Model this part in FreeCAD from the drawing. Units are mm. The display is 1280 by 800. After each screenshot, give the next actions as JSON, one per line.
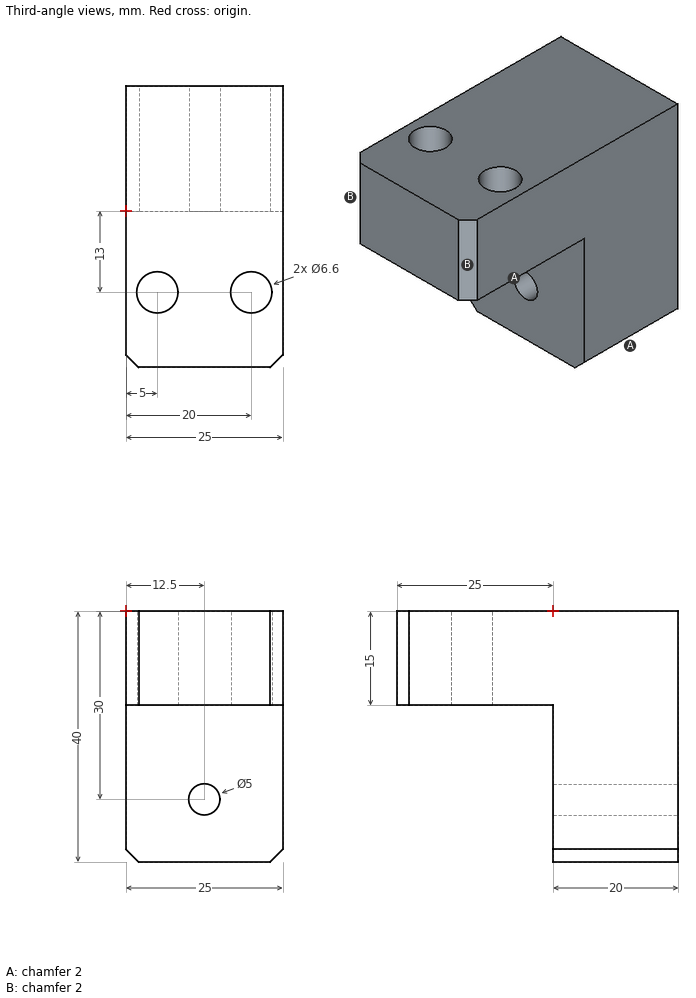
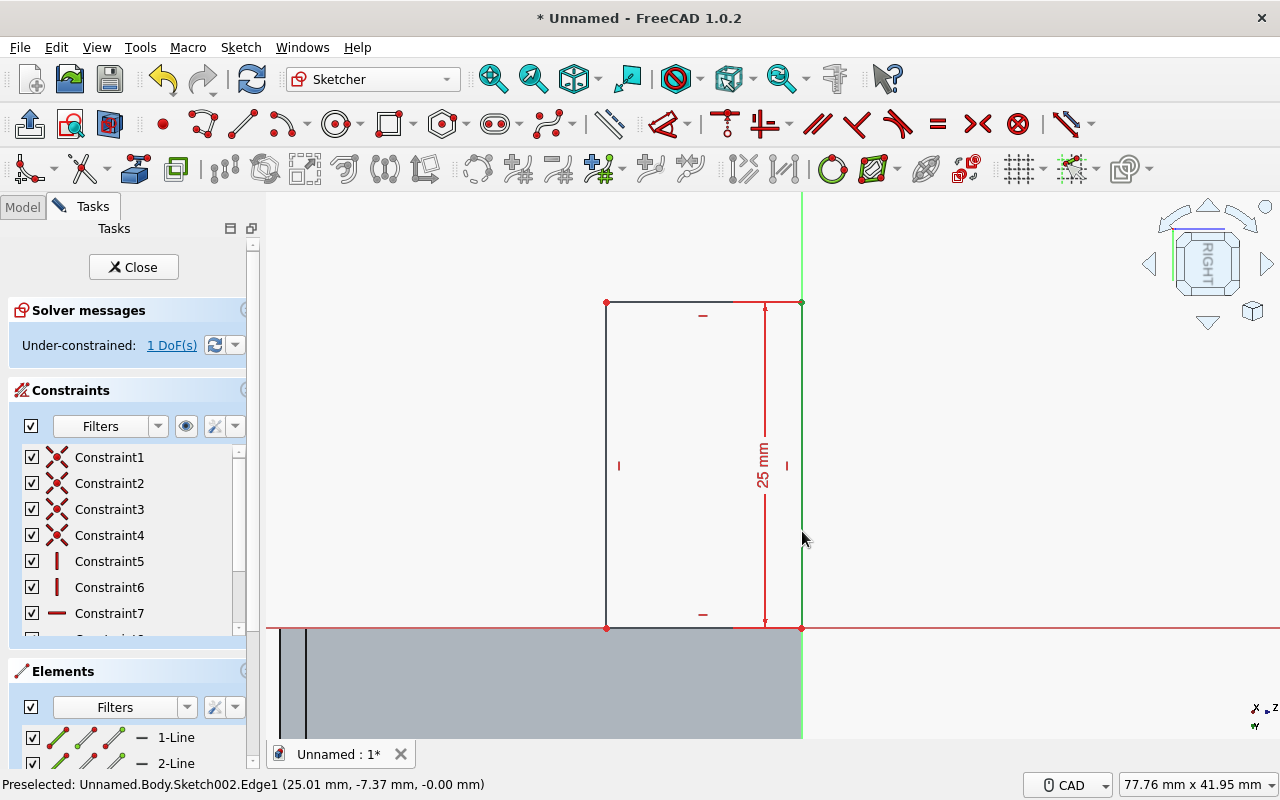
{"action": "left_click", "coordinate": [743, 302]}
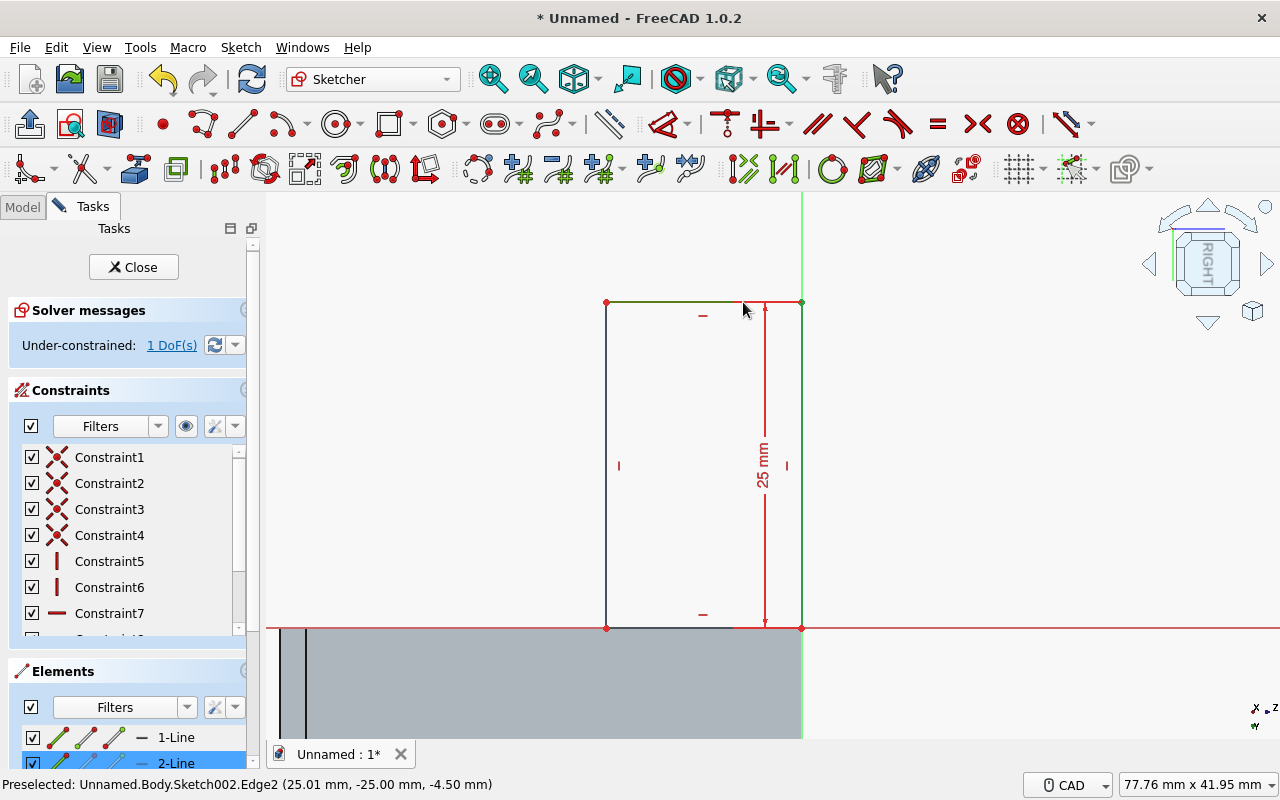
{"action": "left_click", "coordinate": [690, 124]}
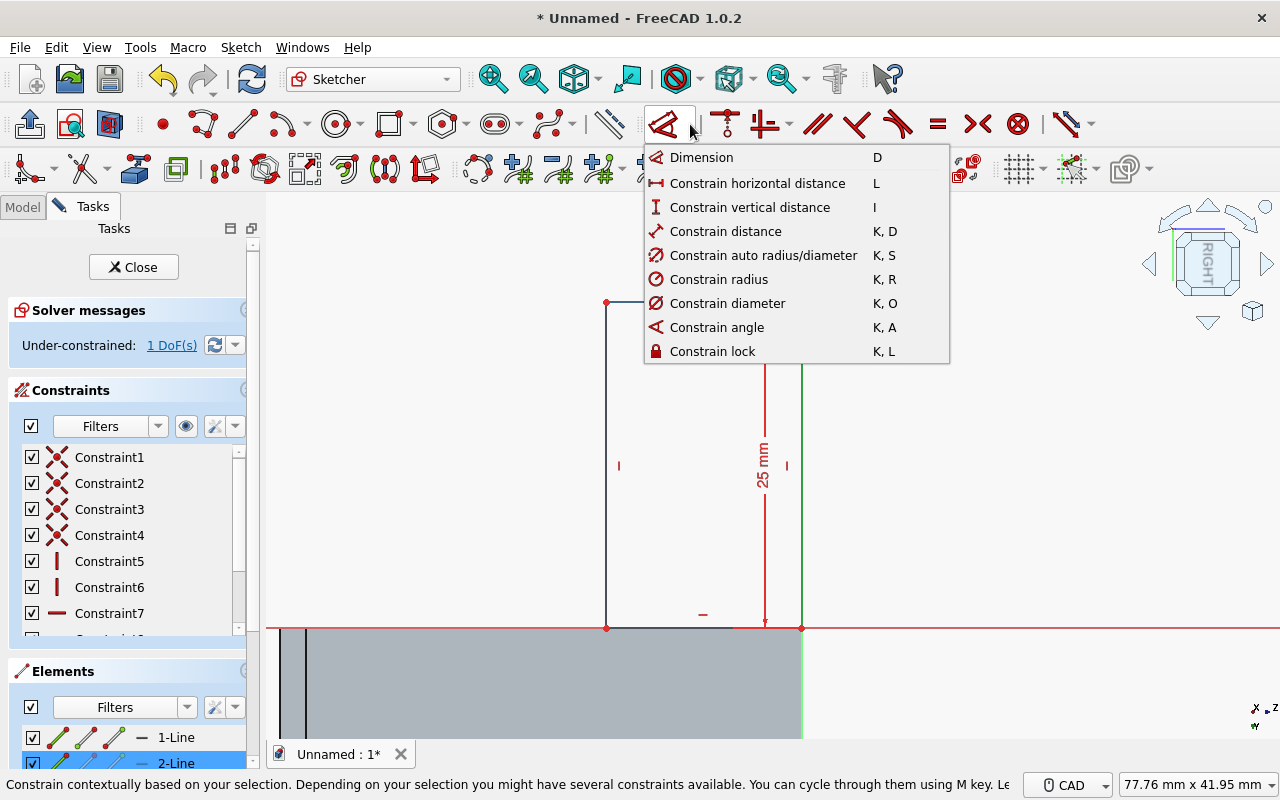
{"action": "left_click", "coordinate": [797, 183]}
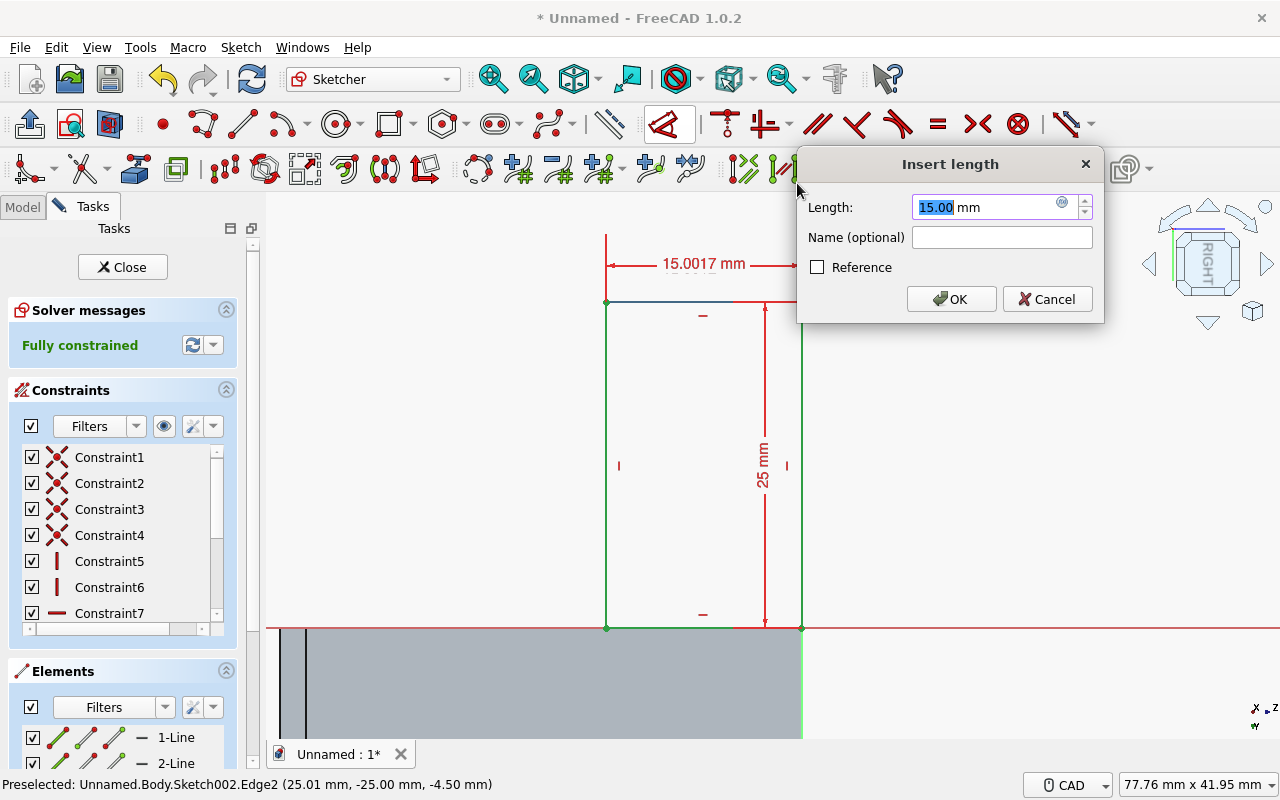
{"action": "type", "text": "15"}
{"action": "key", "text": "Return"}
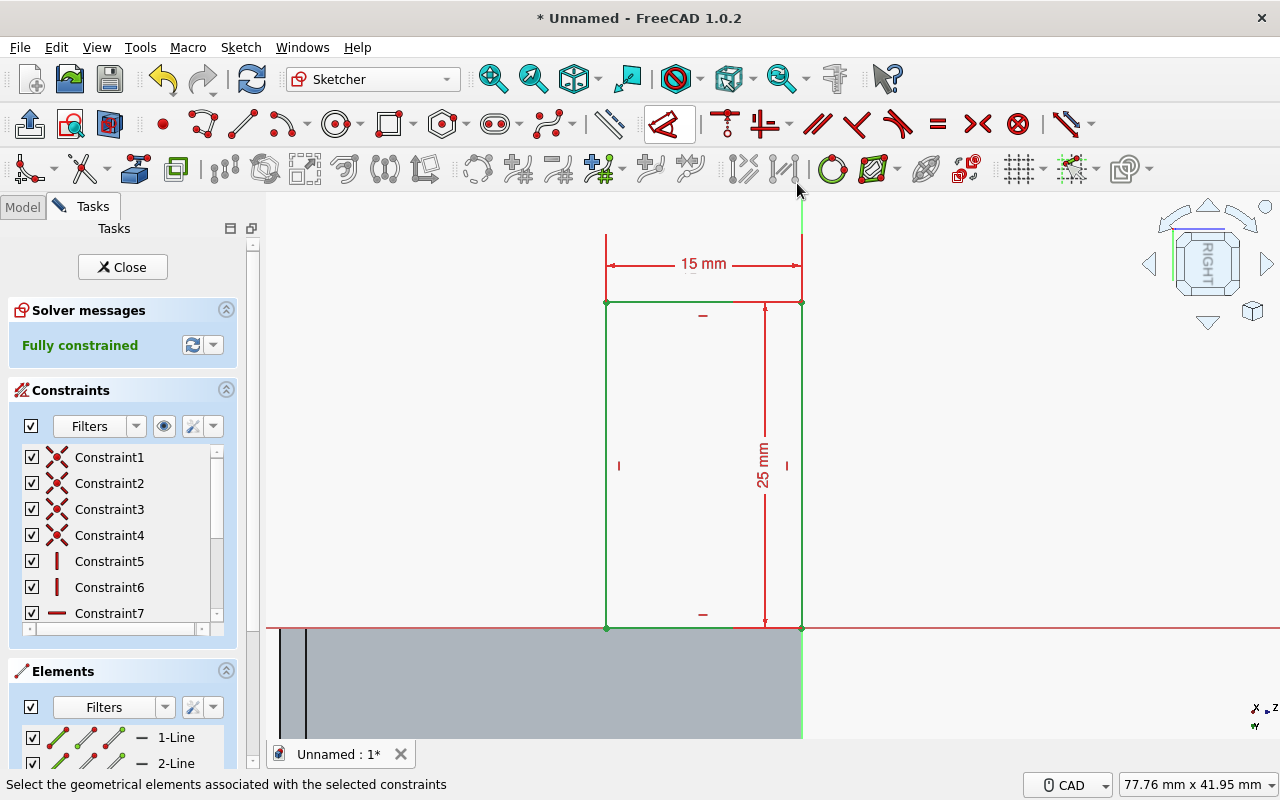
{"action": "left_click", "coordinate": [123, 267]}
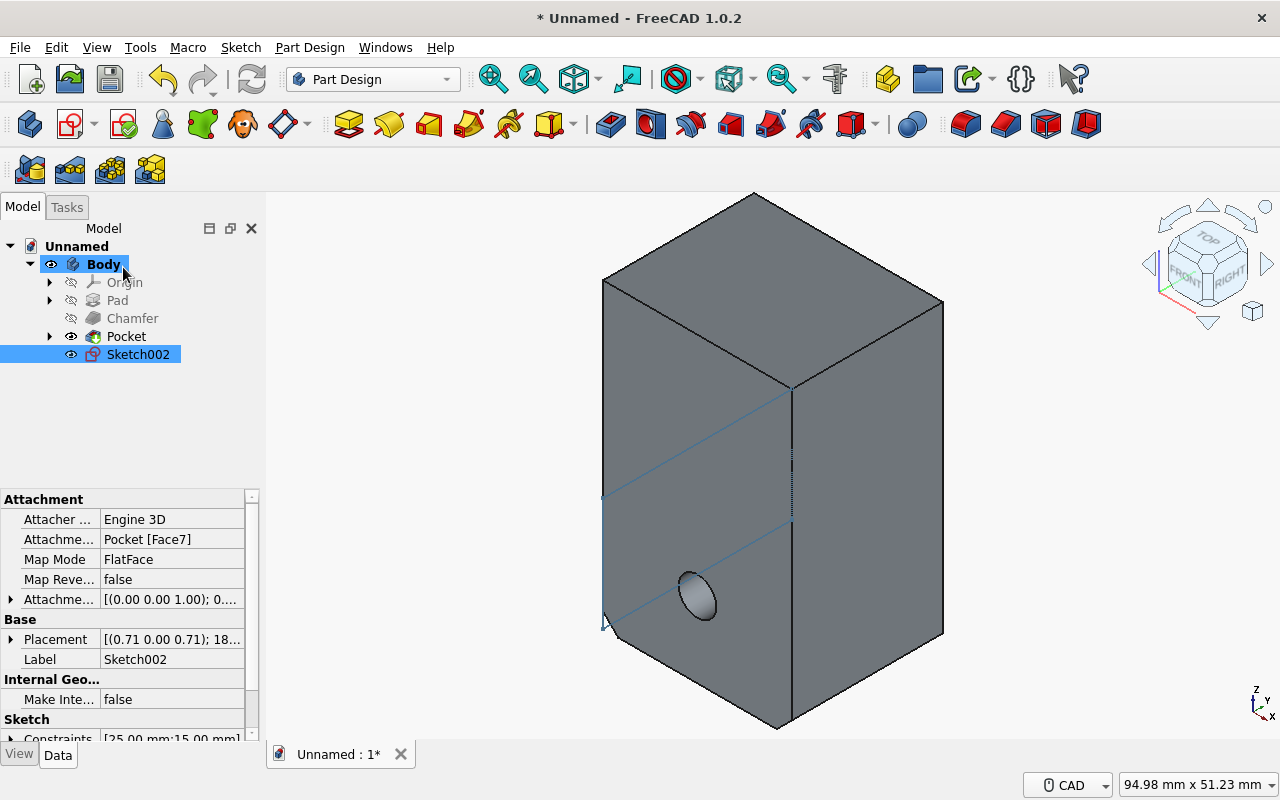
{"action": "left_click", "coordinate": [350, 124]}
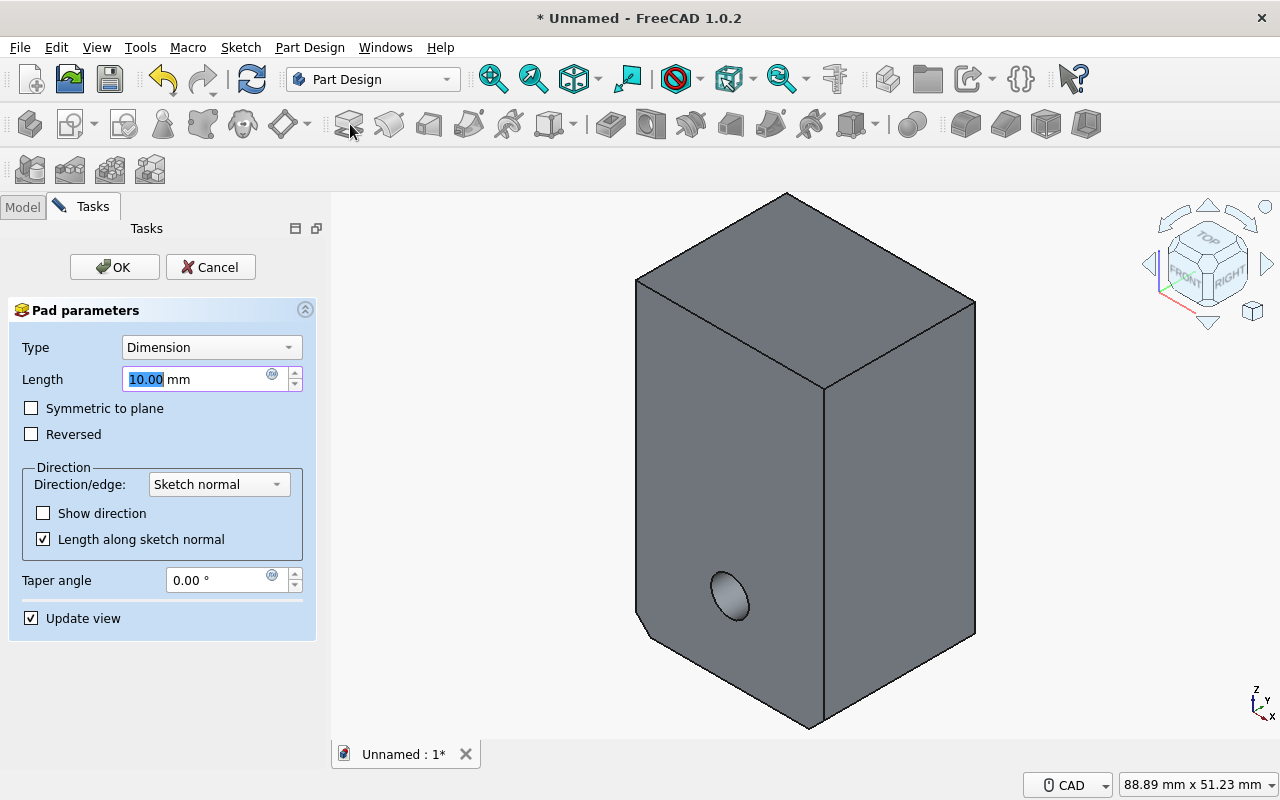
{"action": "type", "text": "25"}
{"action": "key", "text": "Tab"}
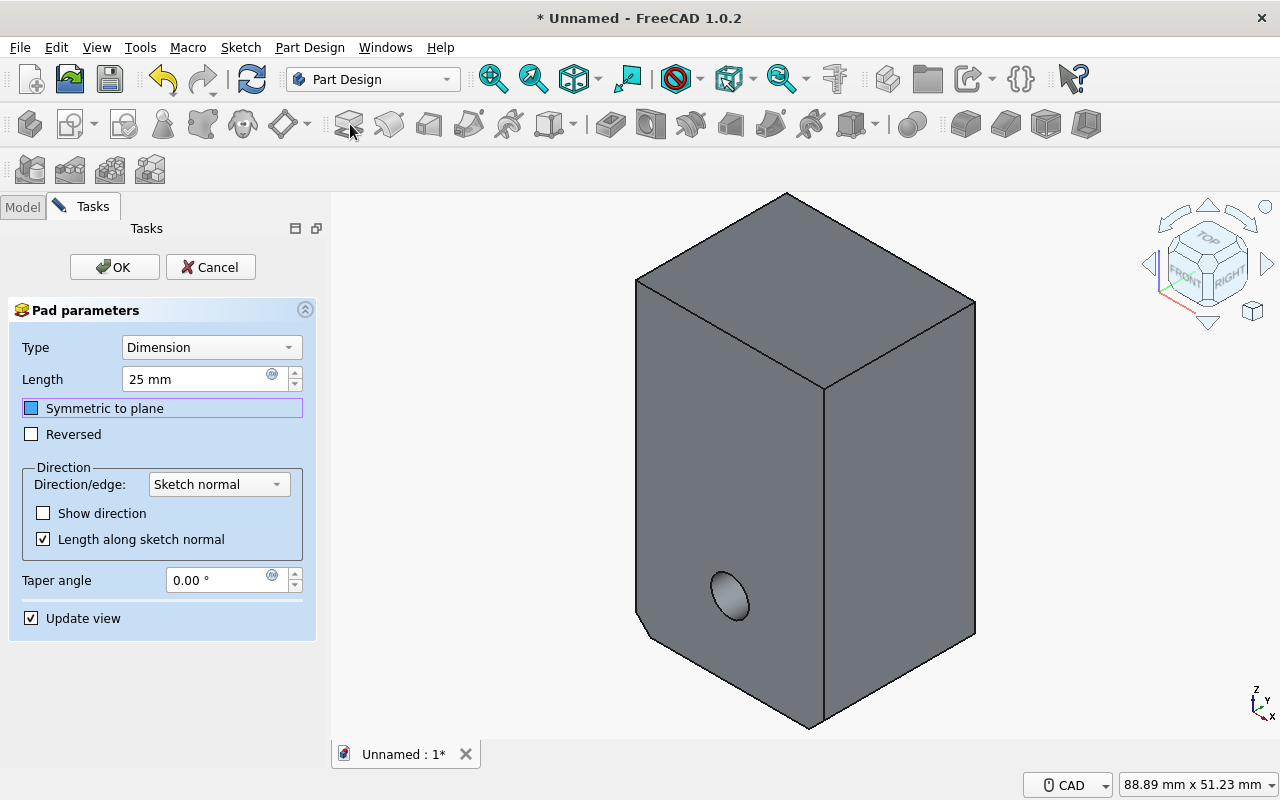
{"action": "left_click", "coordinate": [30, 434]}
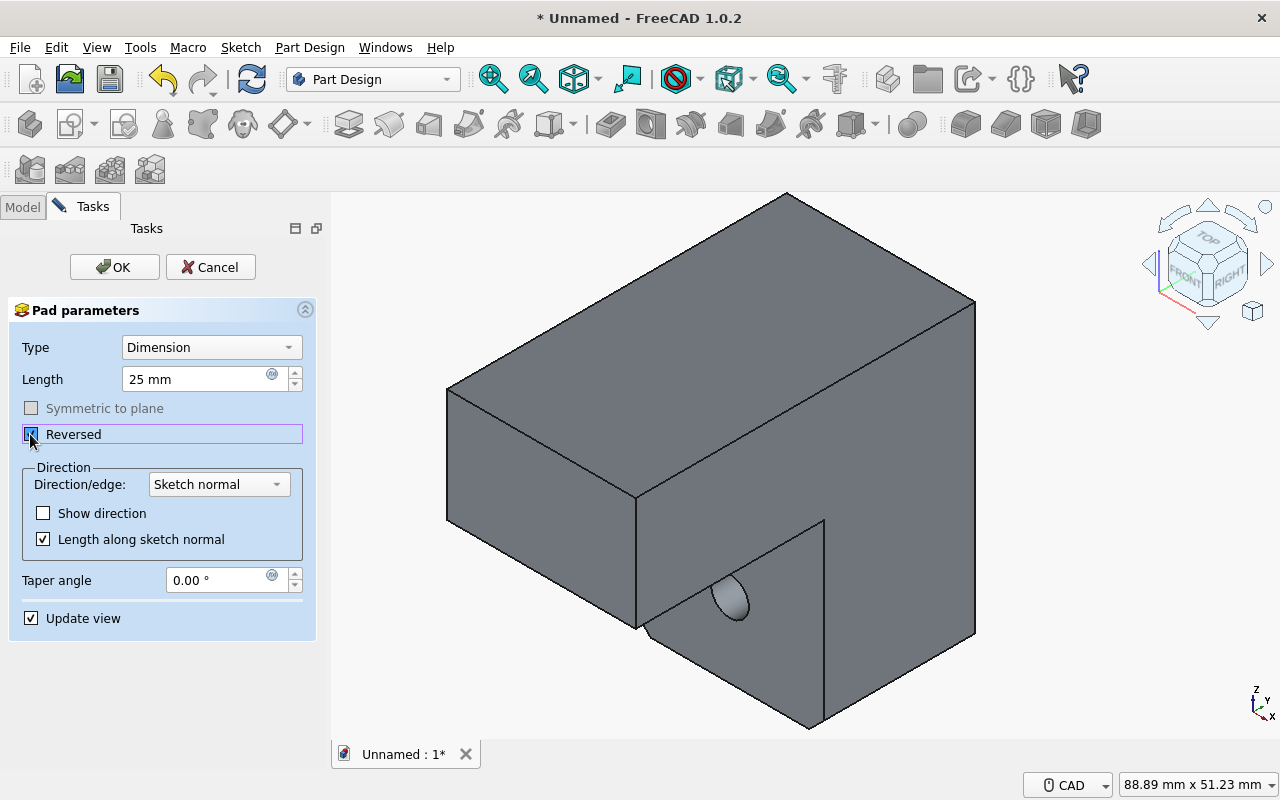
{"action": "left_click", "coordinate": [115, 267]}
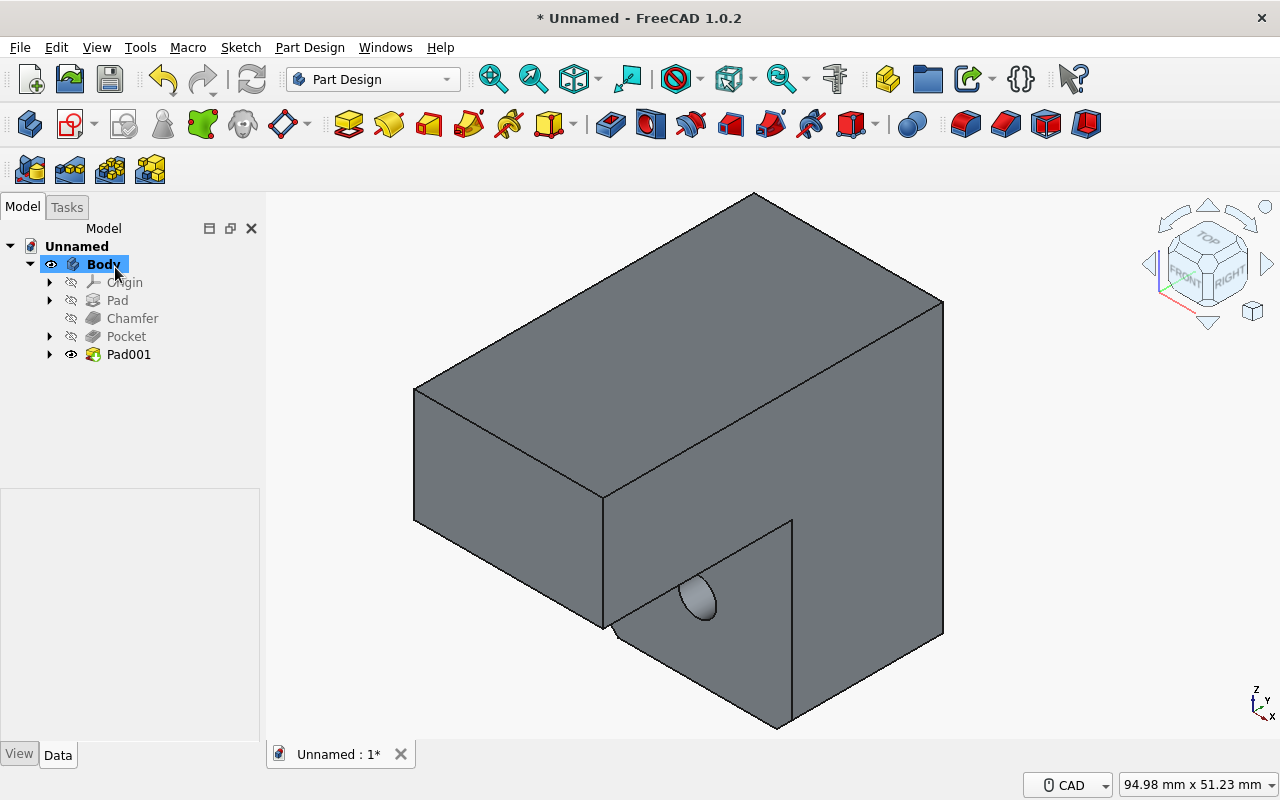
{"action": "left_click", "coordinate": [494, 80]}